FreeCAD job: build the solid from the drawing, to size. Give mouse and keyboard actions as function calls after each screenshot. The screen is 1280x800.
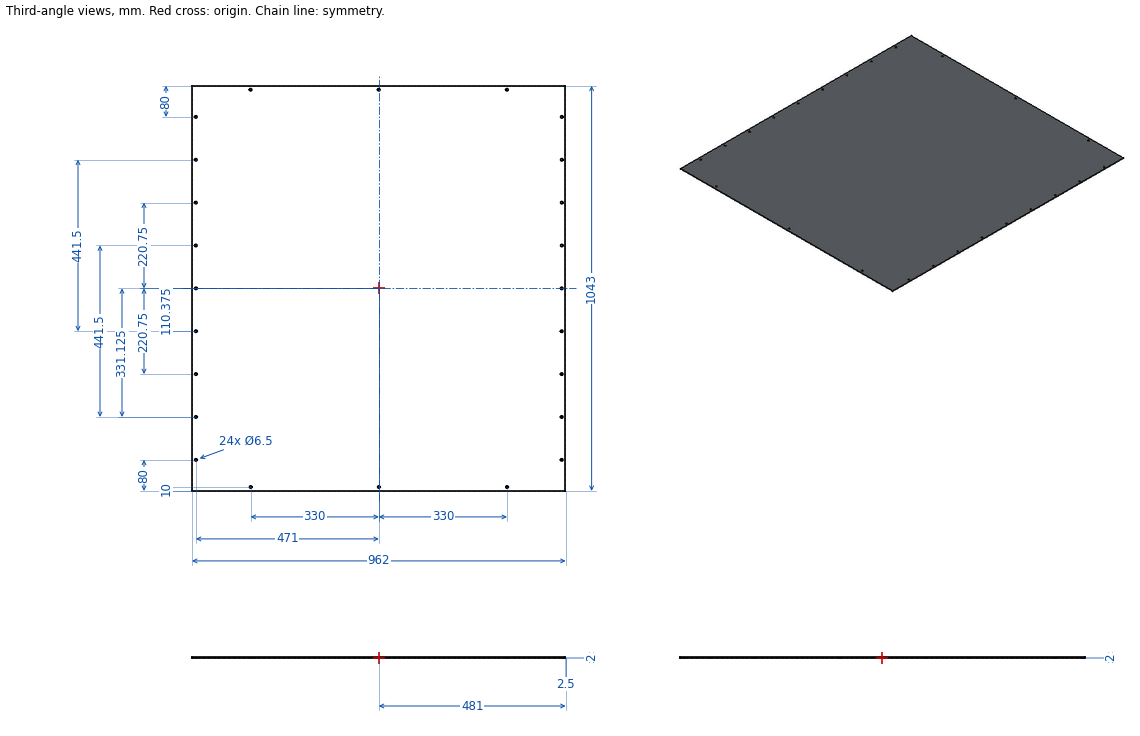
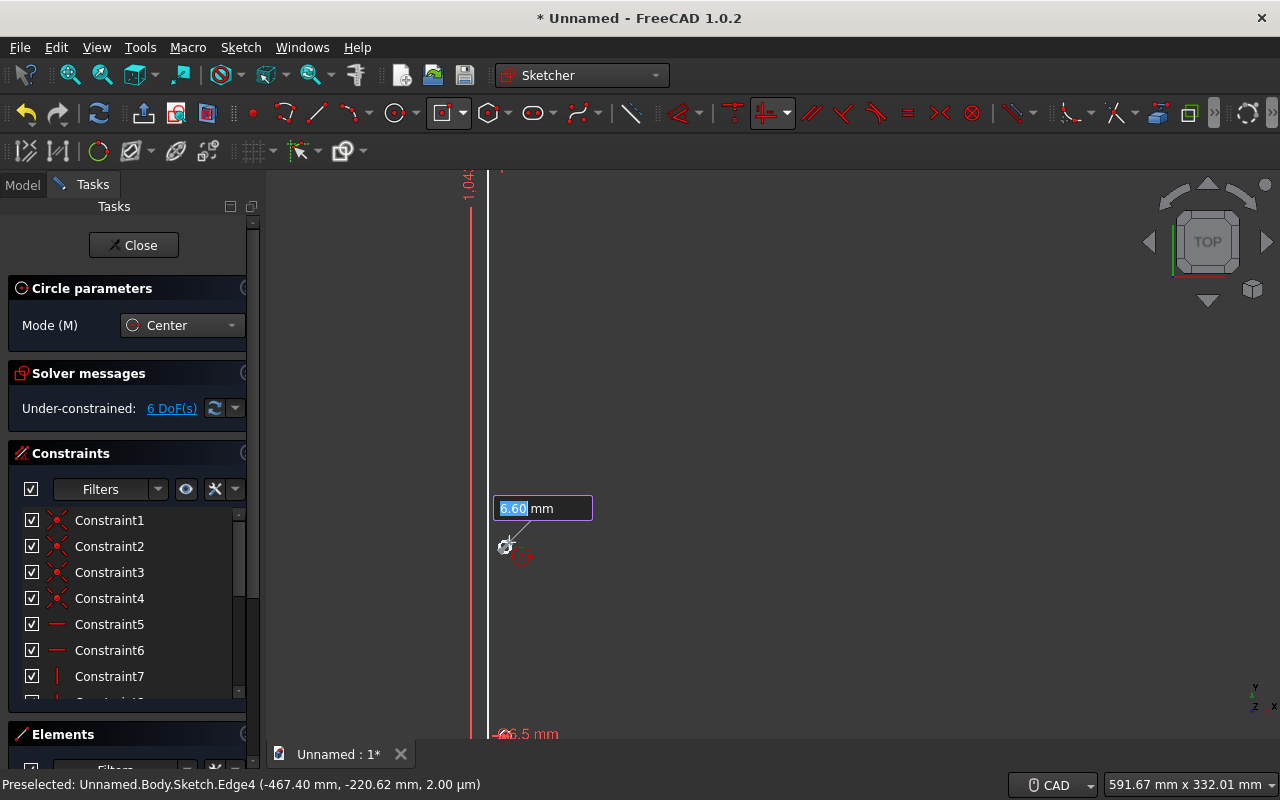
text(6.5)
key(Return)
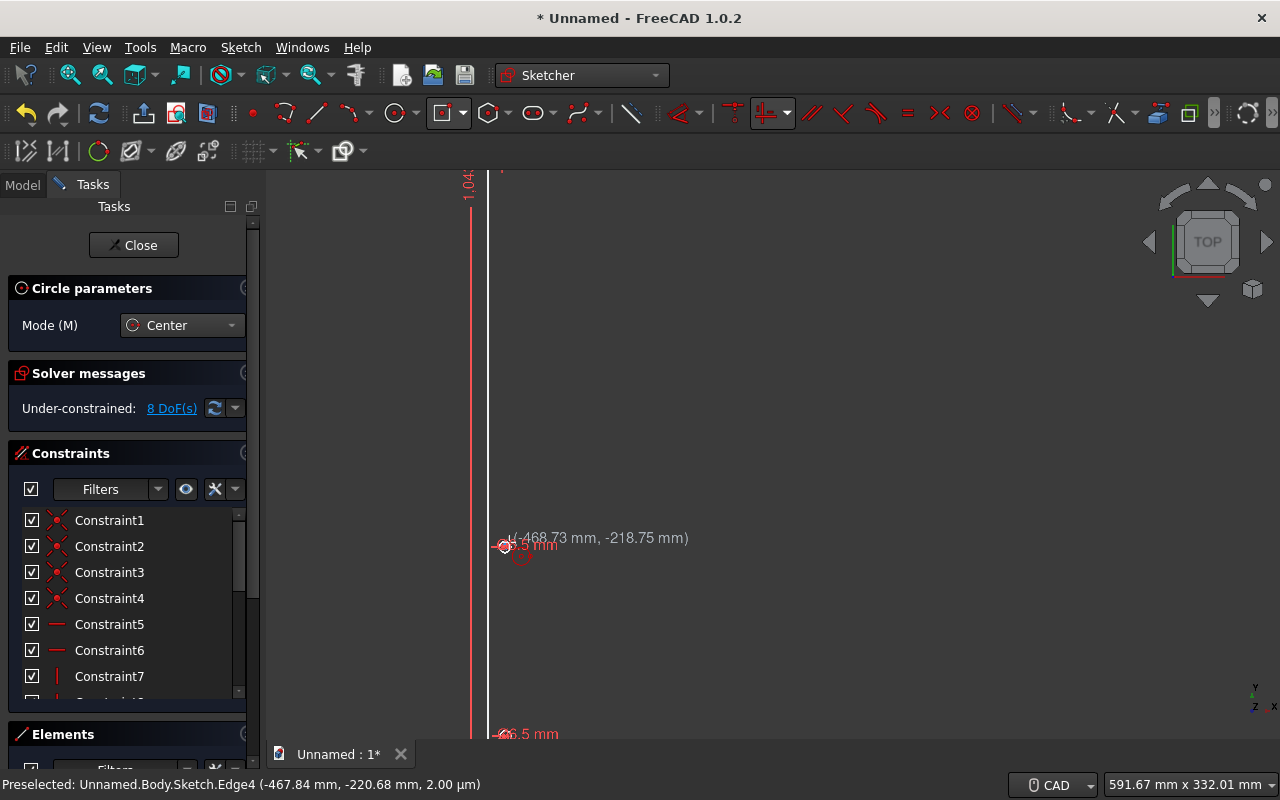
scroll(505, 357, up, 8)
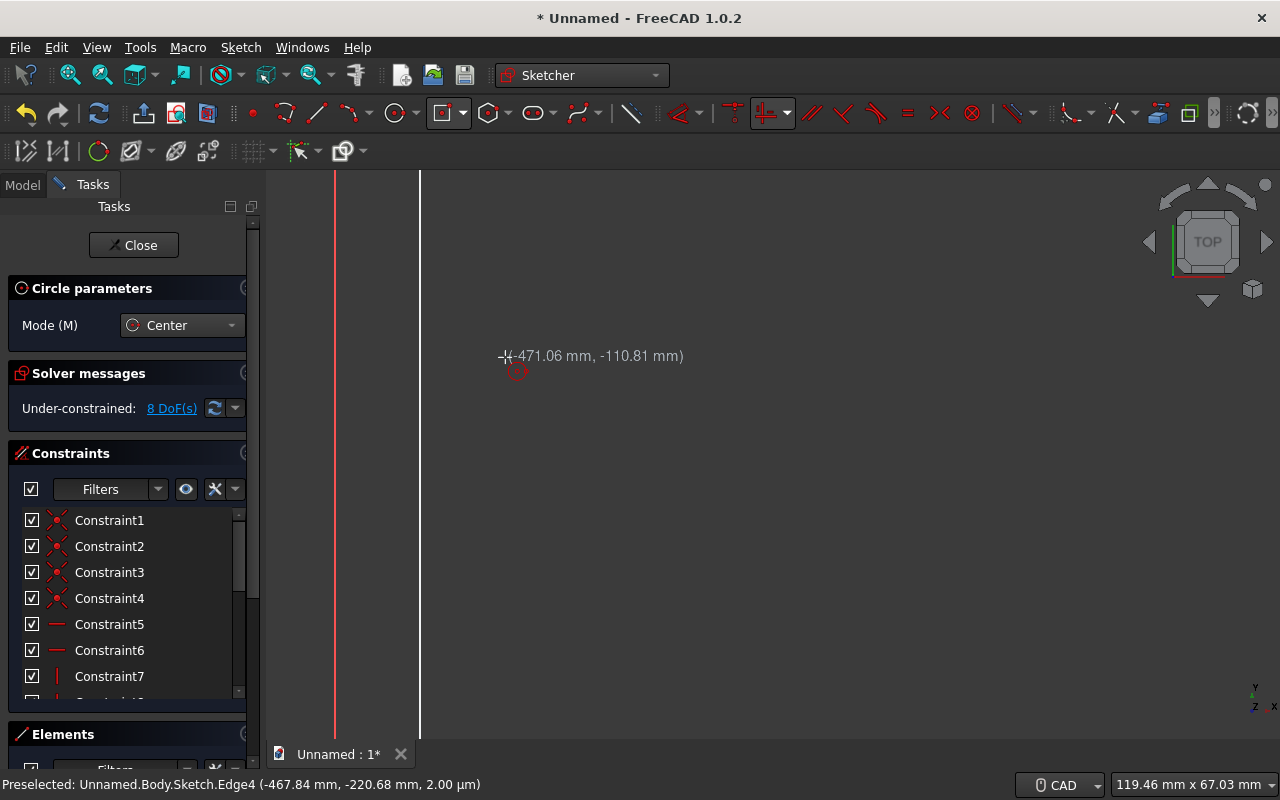
scroll(505, 509, down, 15)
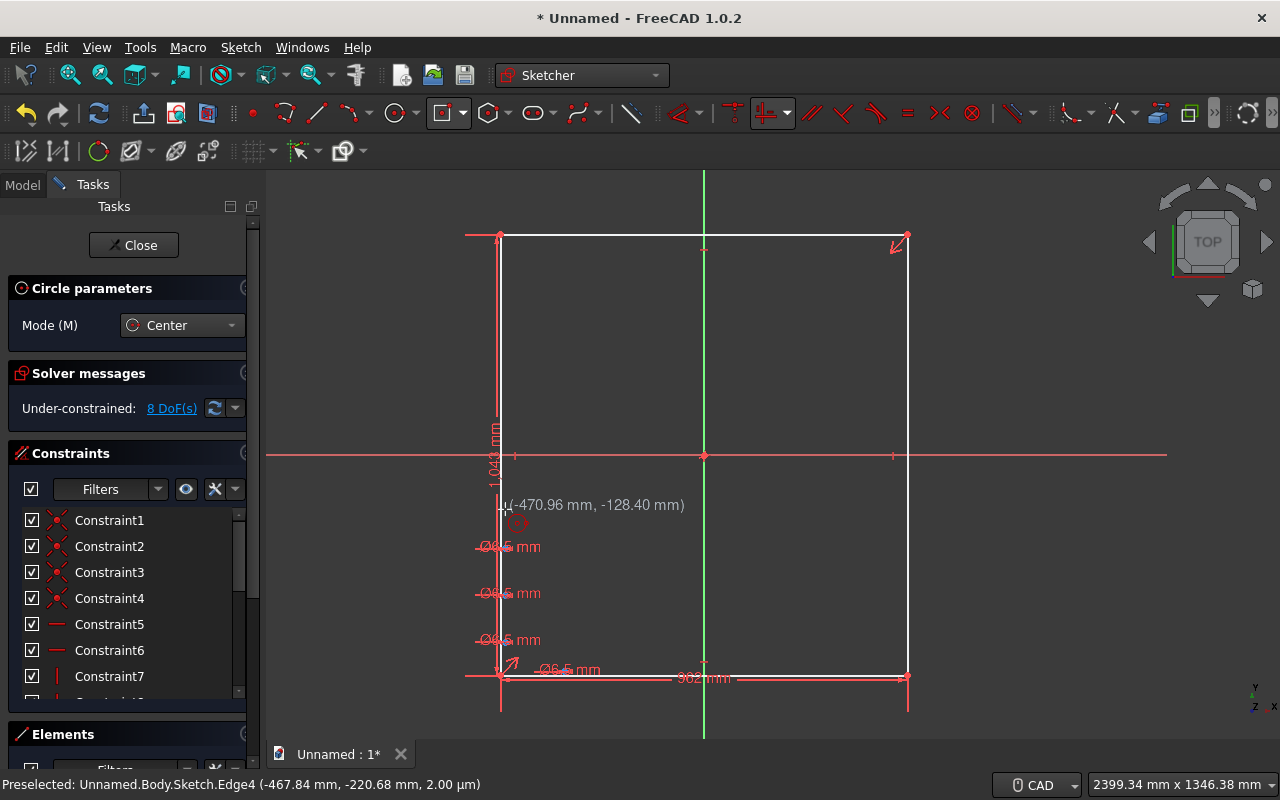
scroll(505, 502, up, 7)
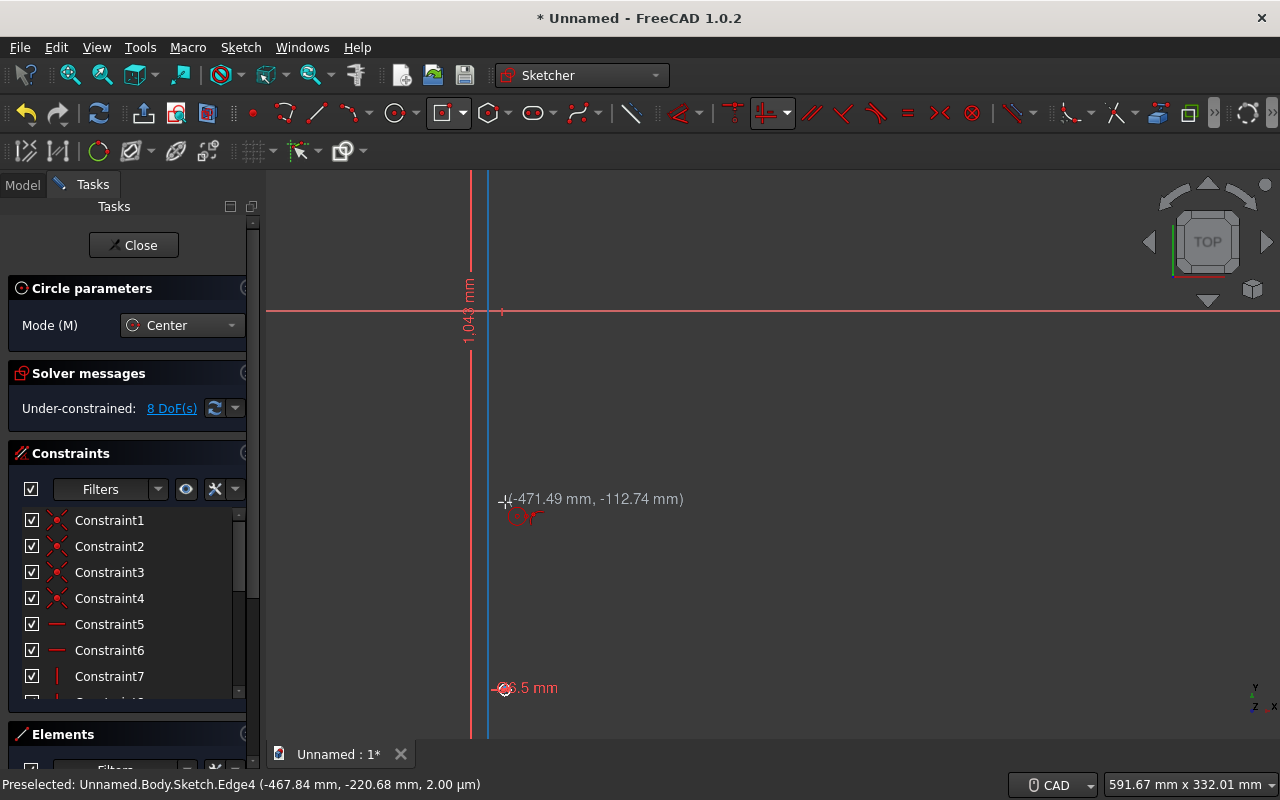
click(505, 500)
move(509, 496)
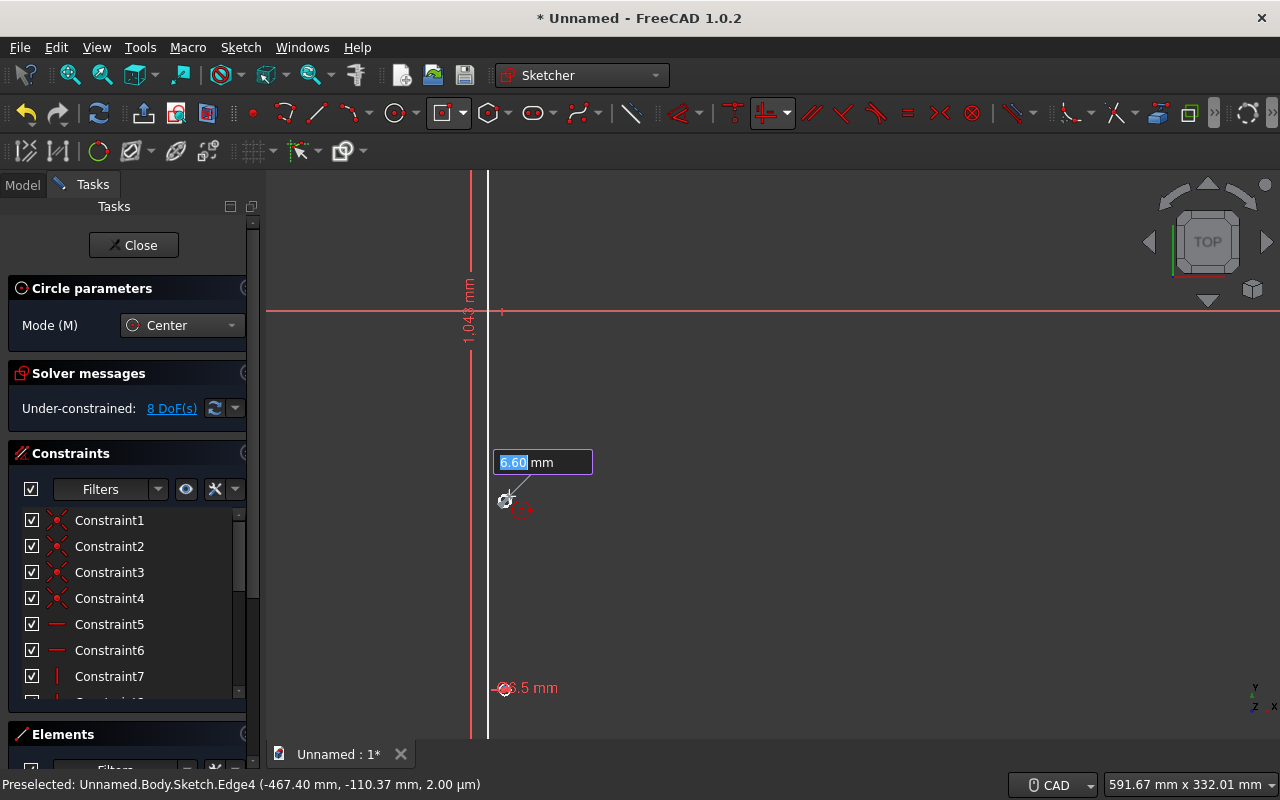
text(6.5)
key(Return)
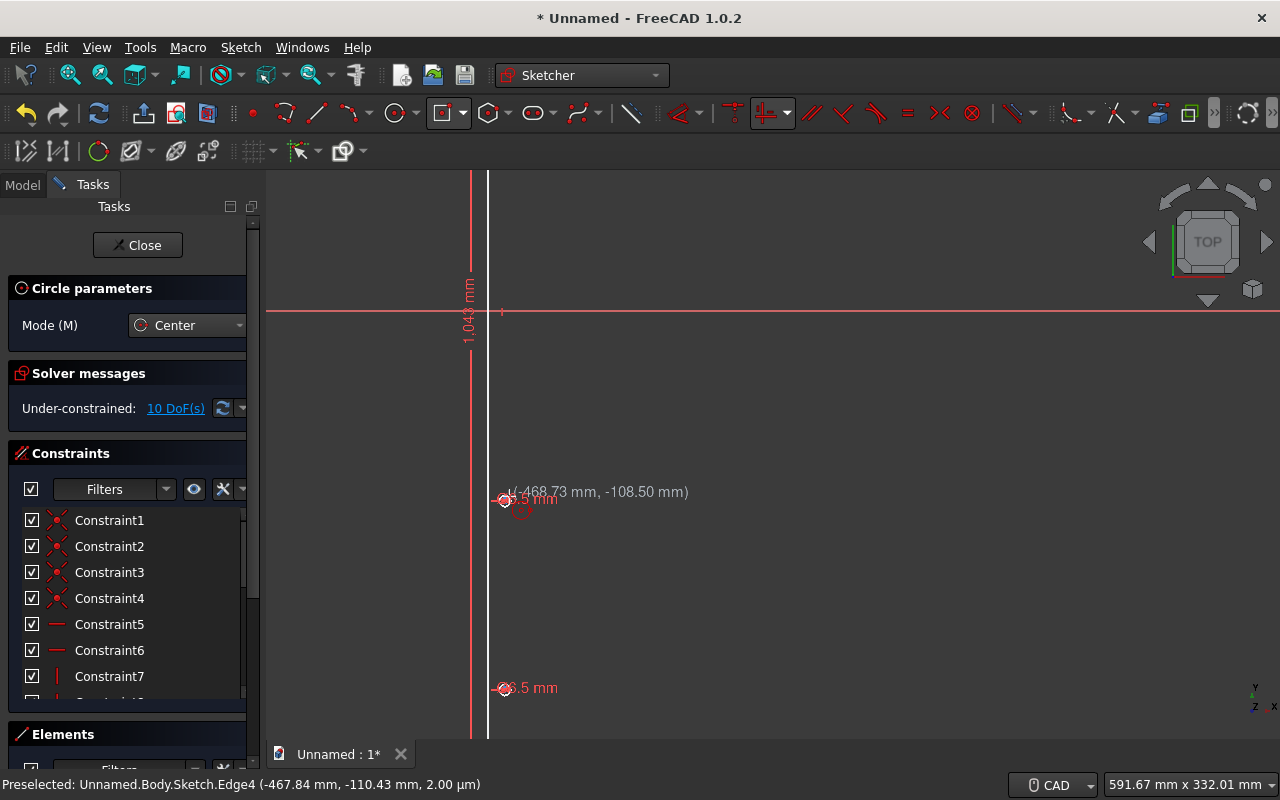
scroll(551, 491, down, 8)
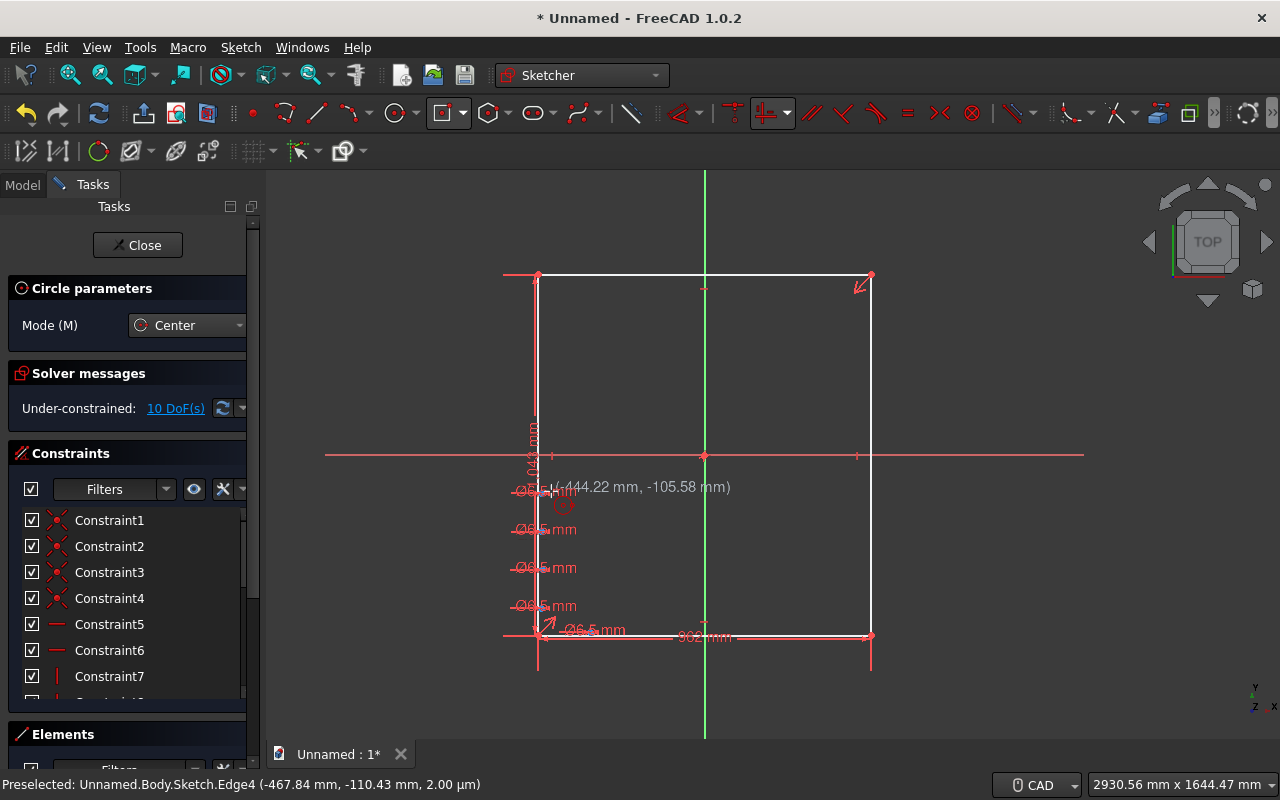
scroll(705, 632, up, 16)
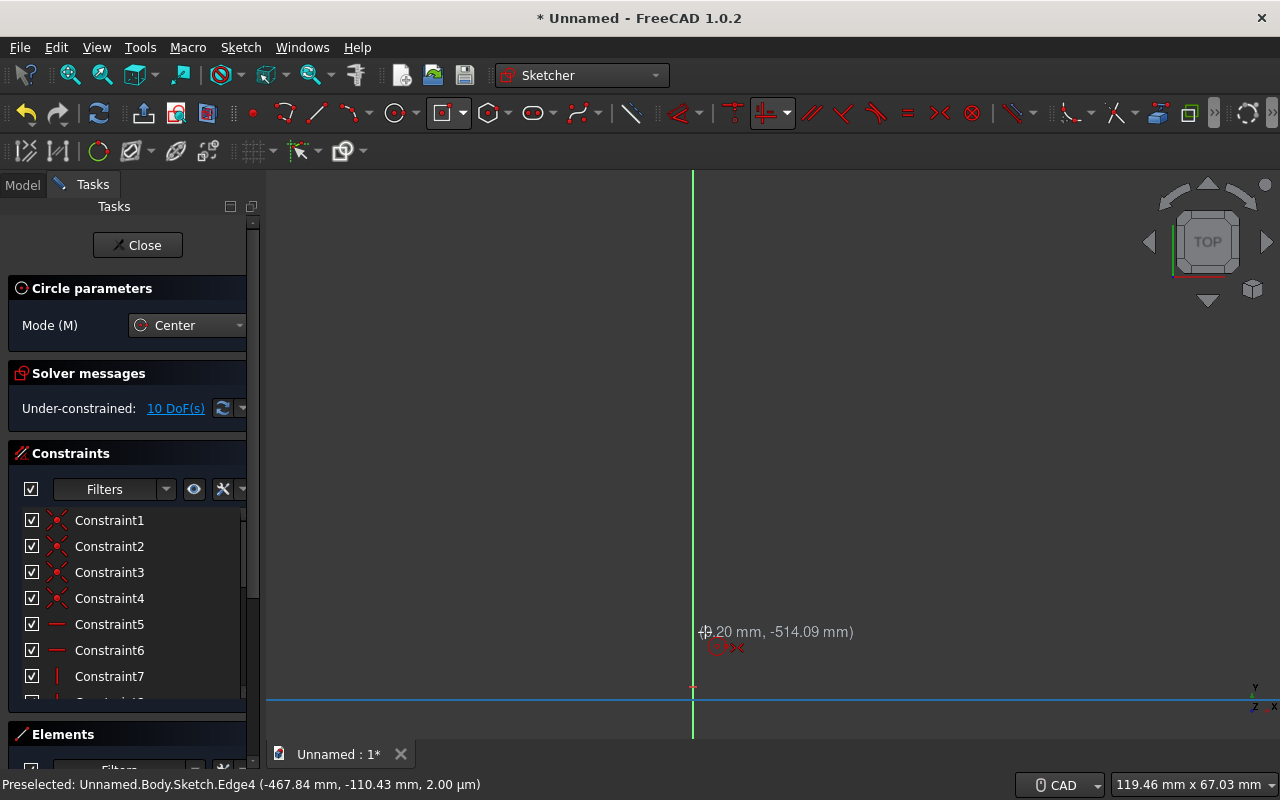
scroll(705, 674, down, 15)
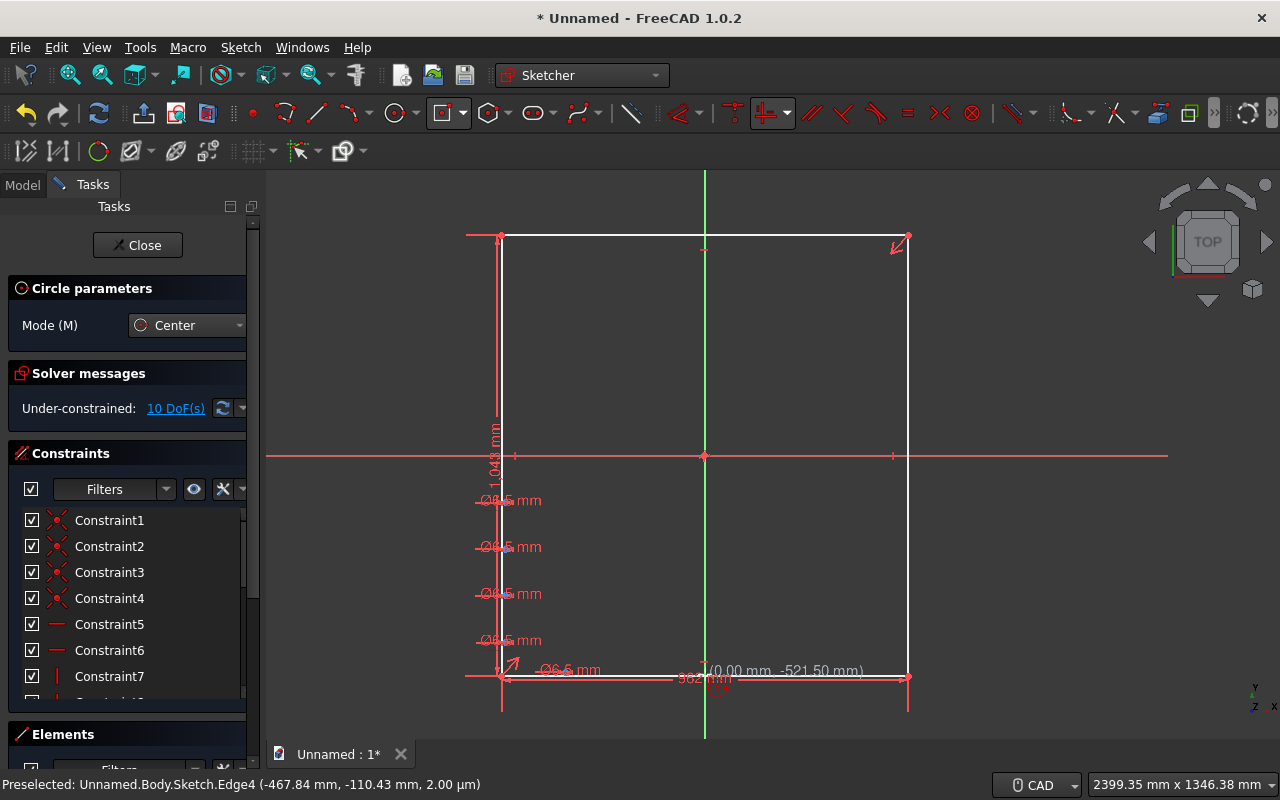
scroll(705, 672, up, 7)